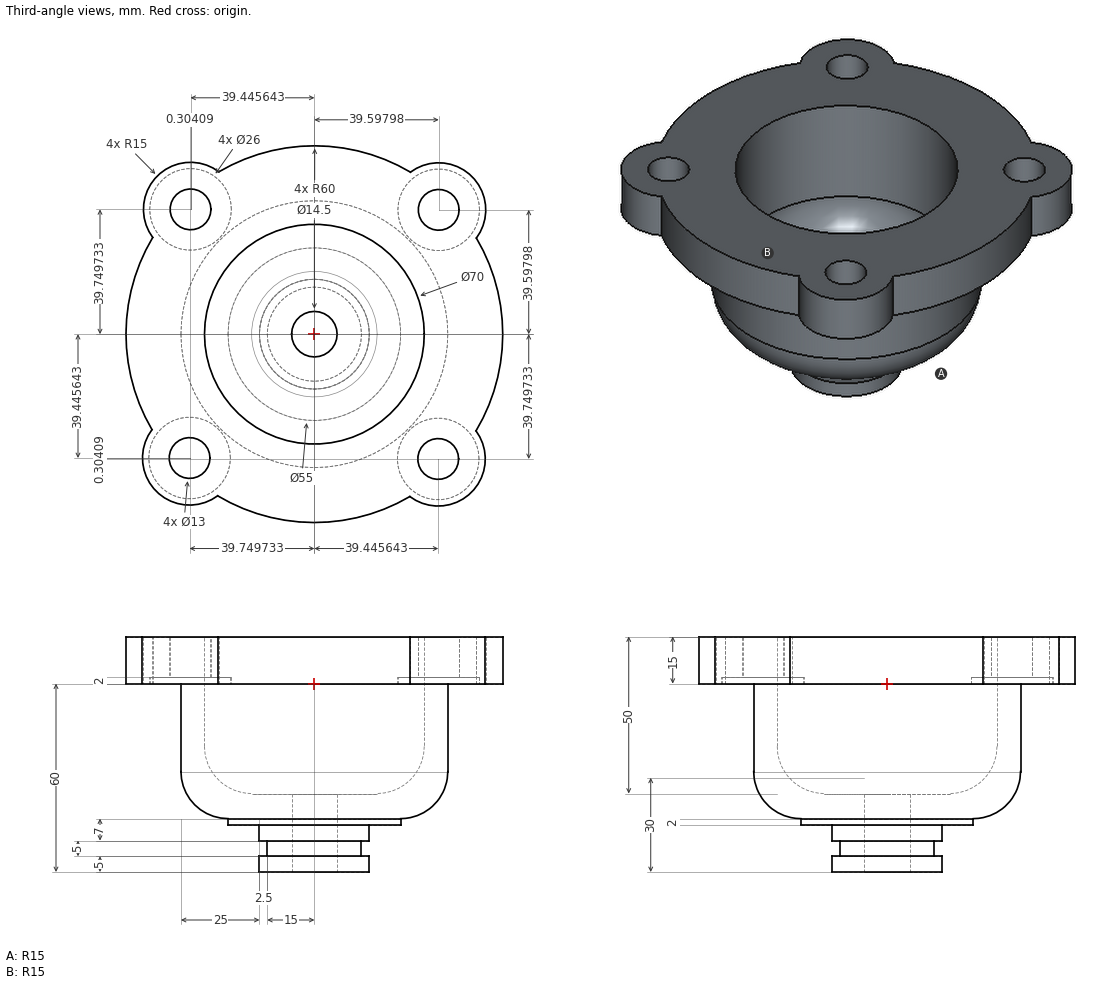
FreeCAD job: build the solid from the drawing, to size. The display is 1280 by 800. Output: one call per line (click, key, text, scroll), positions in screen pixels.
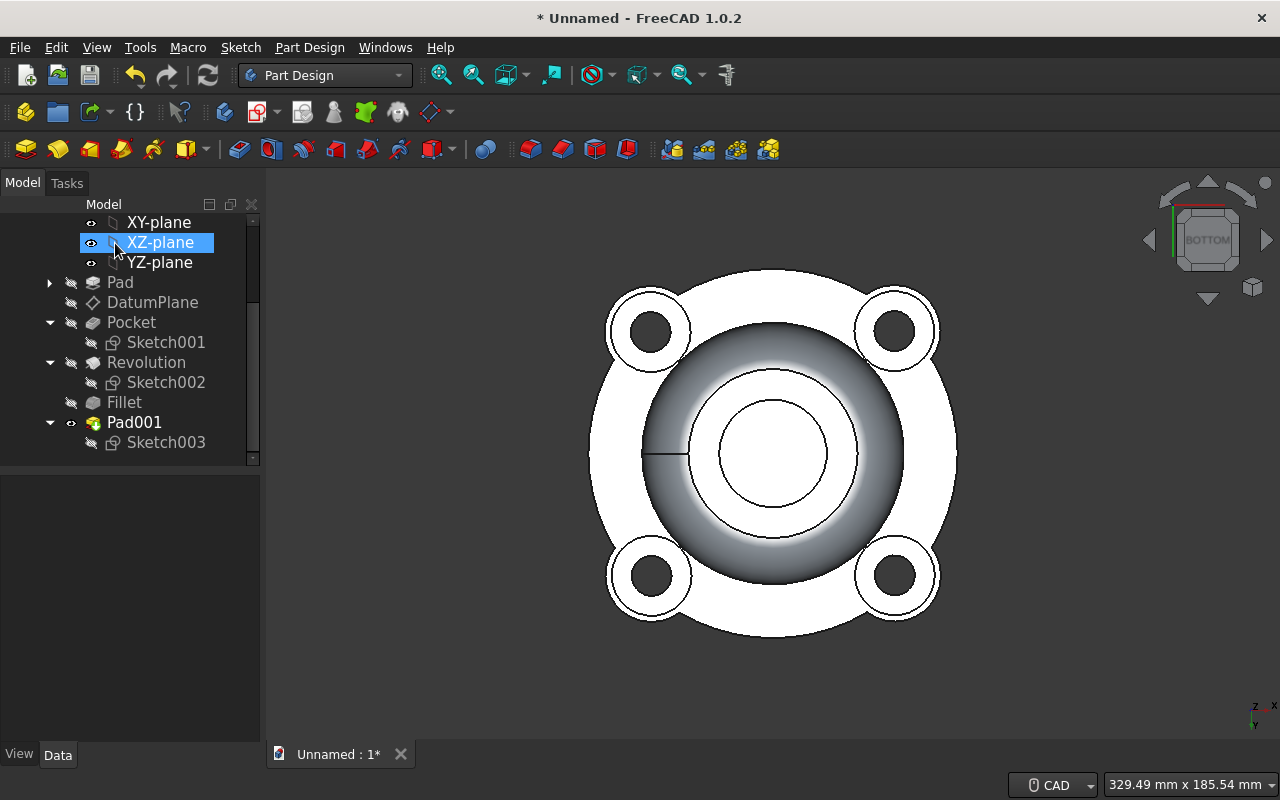
click(773, 452)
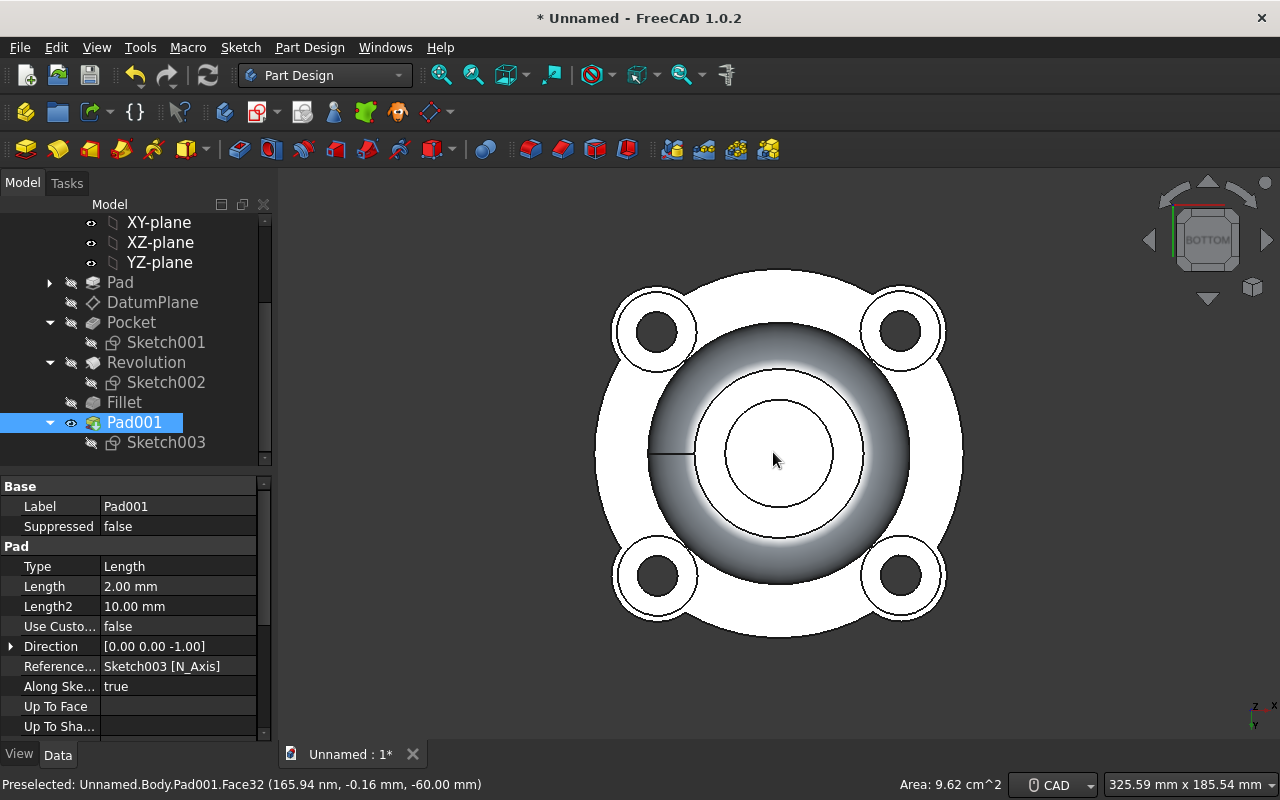
click(258, 112)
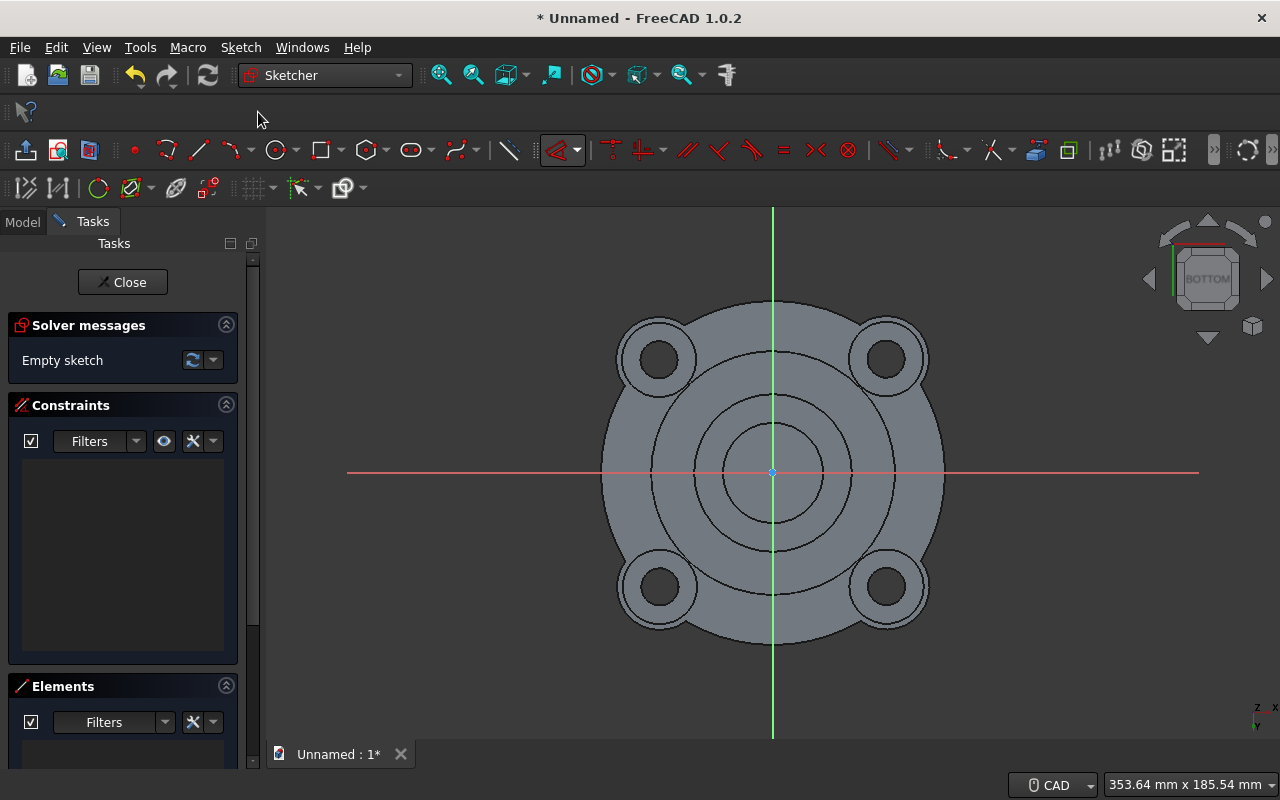
scroll(784, 473, up, 10)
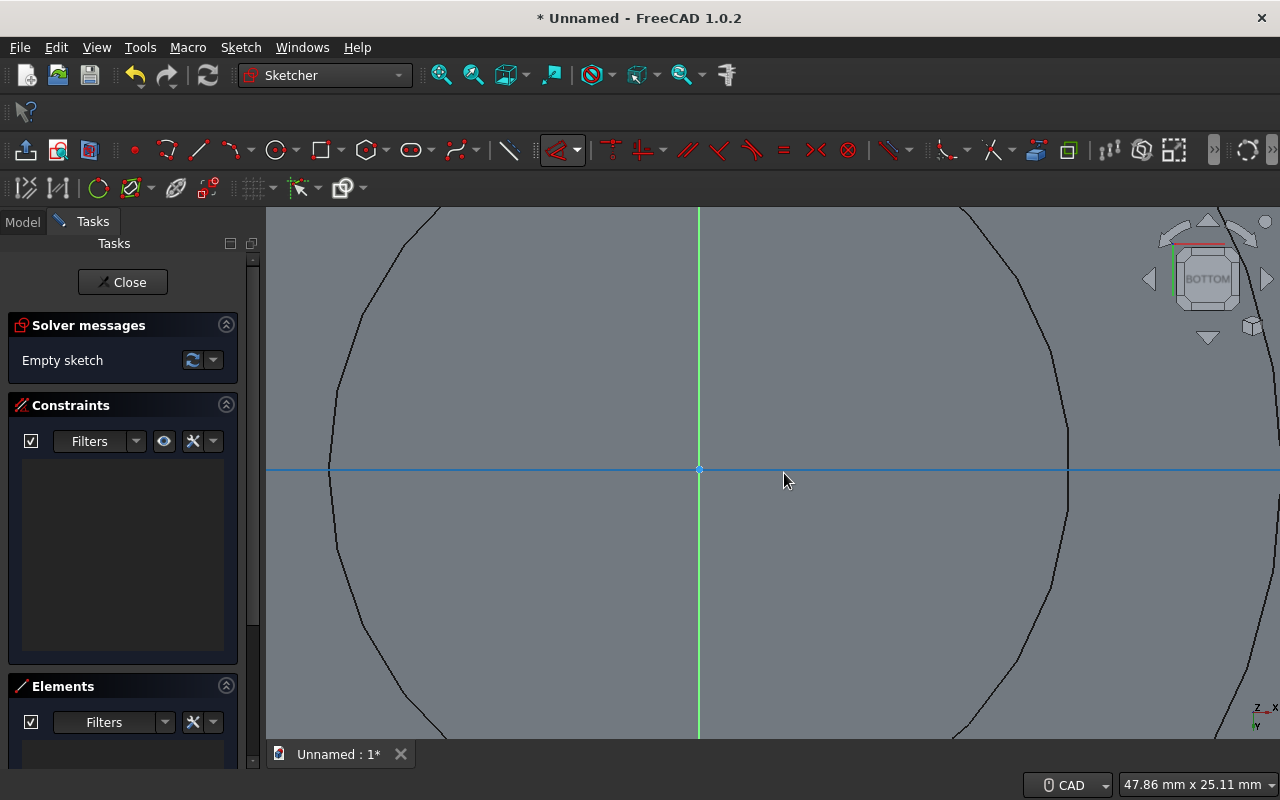
key(g)
key(c)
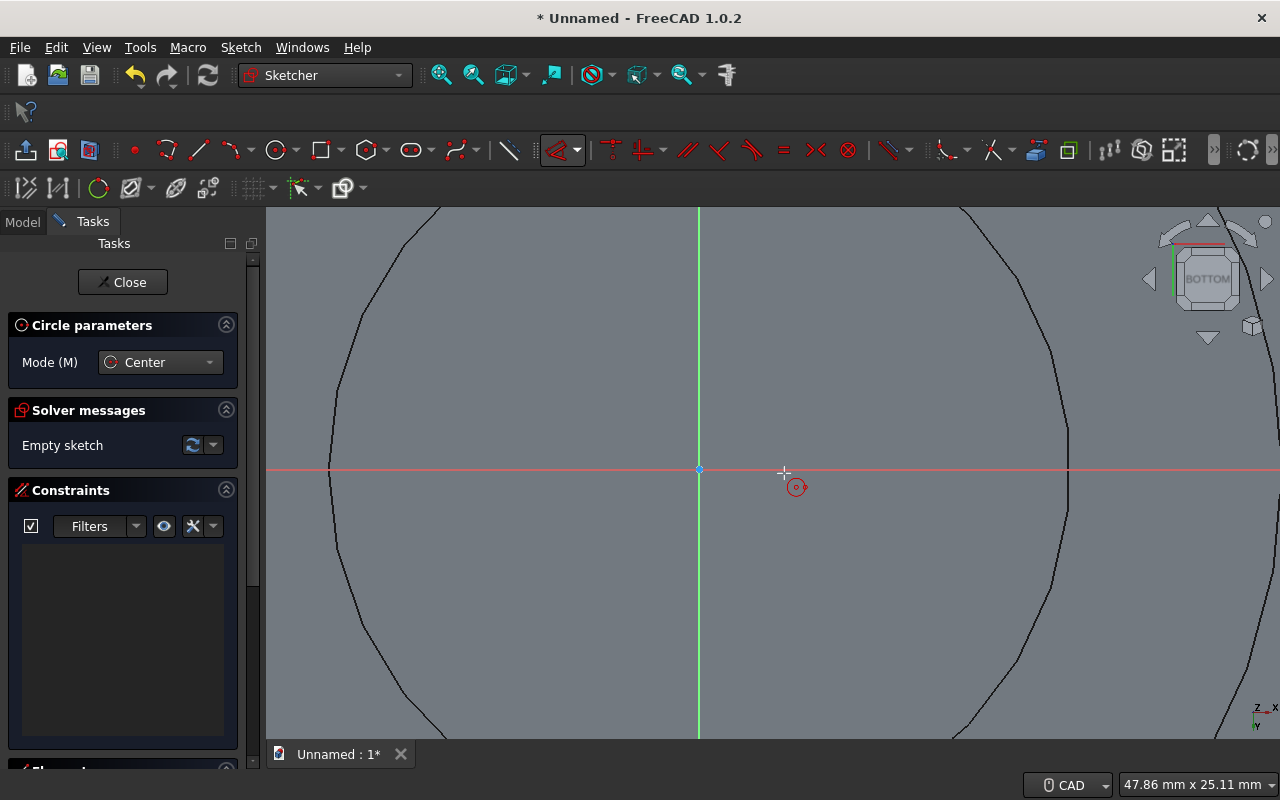
click(699, 470)
move(808, 361)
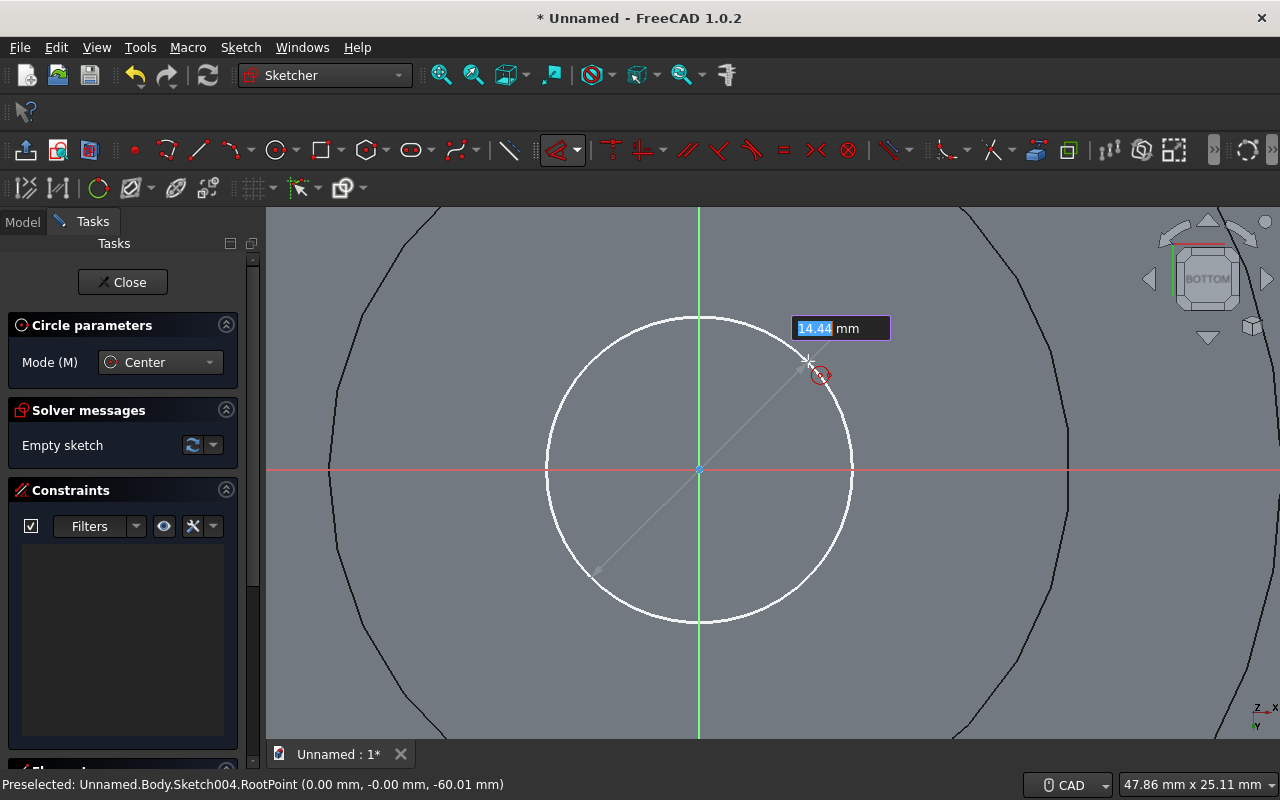
text(14.5)
key(Return)
key(Escape)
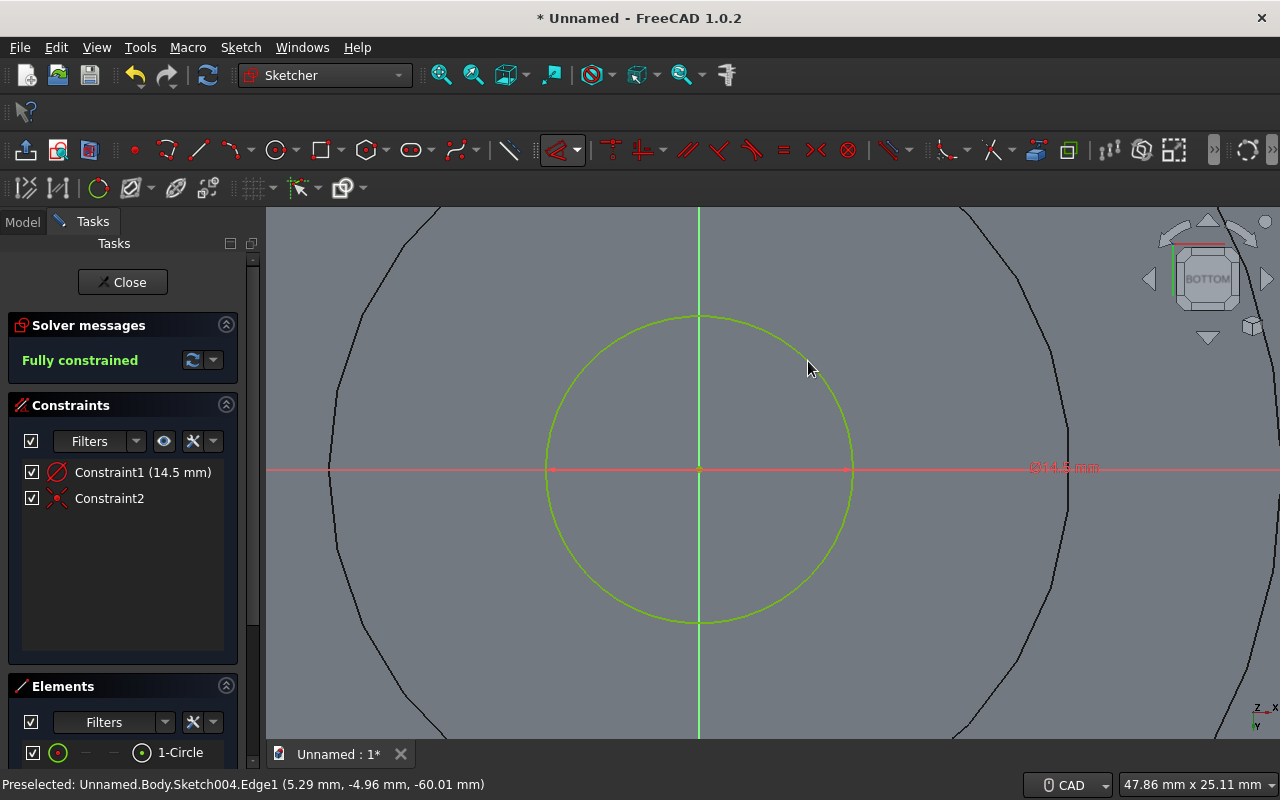
click(123, 282)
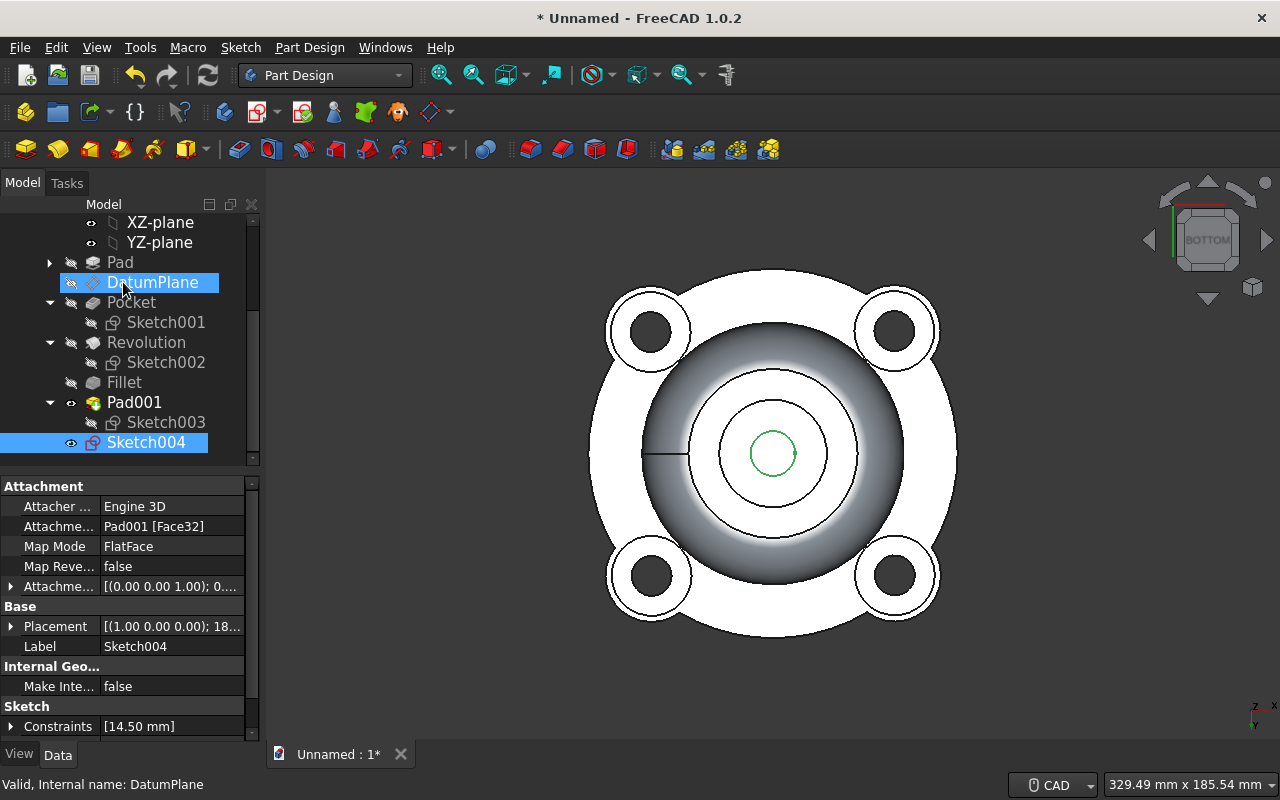
click(240, 150)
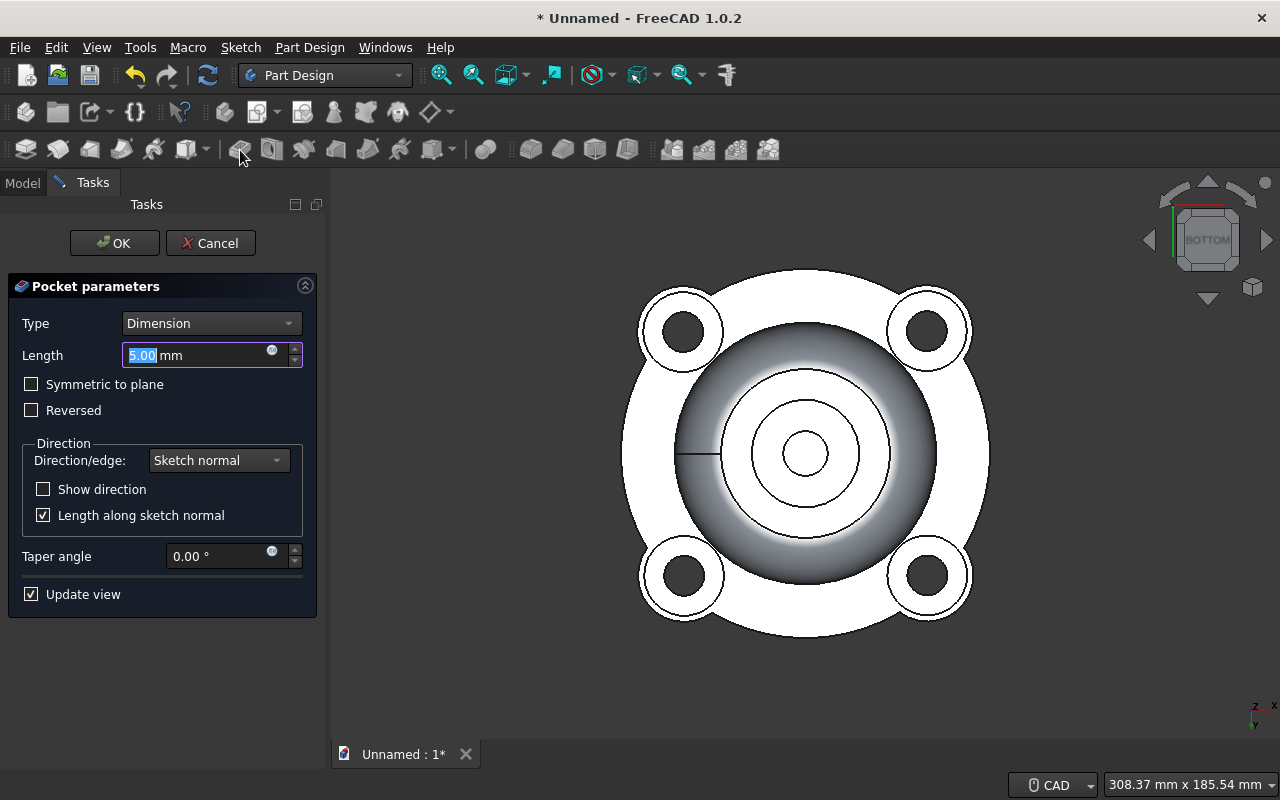
text(30)
key(Tab)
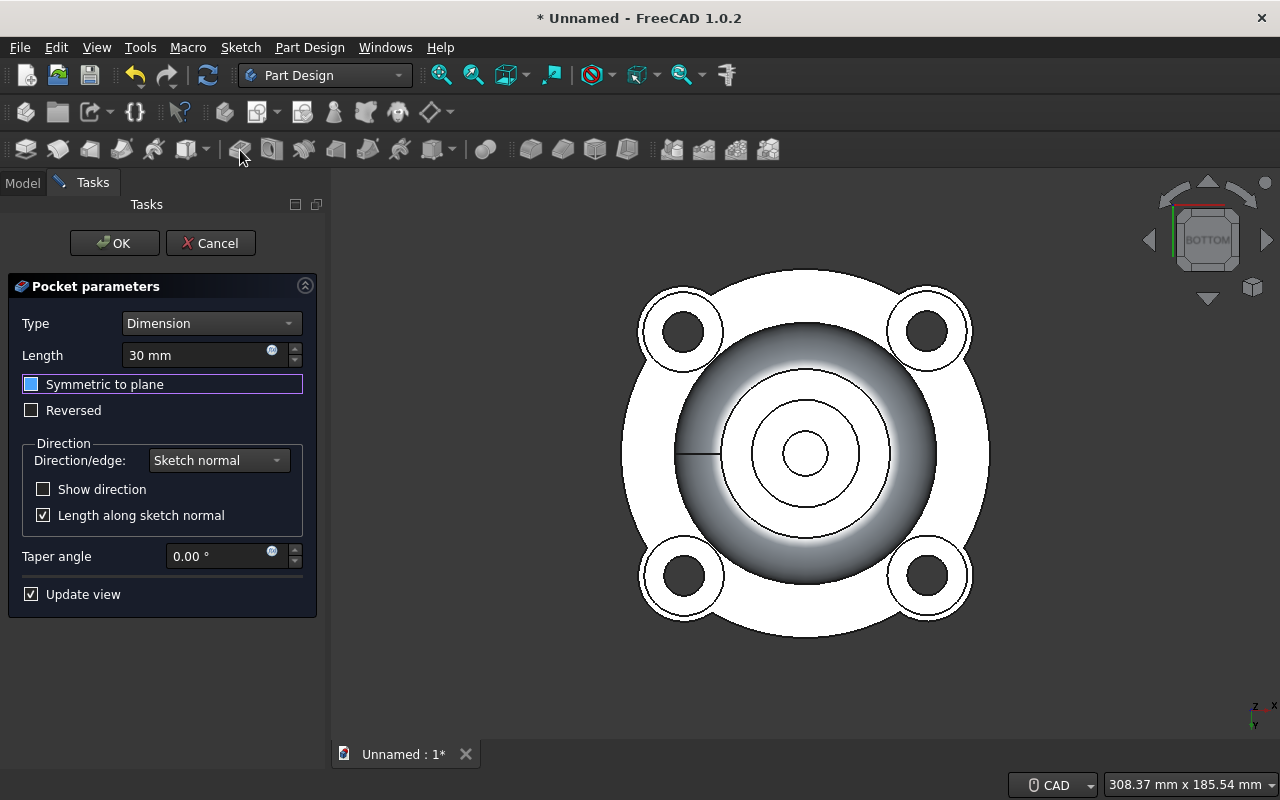
click(115, 243)